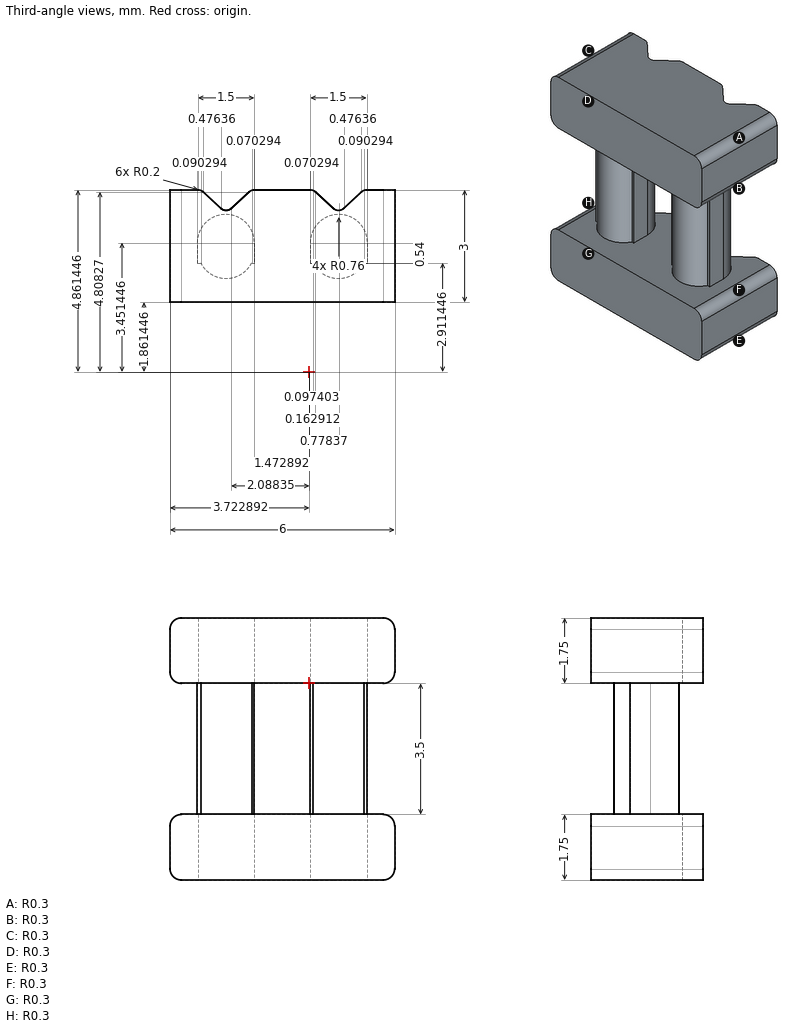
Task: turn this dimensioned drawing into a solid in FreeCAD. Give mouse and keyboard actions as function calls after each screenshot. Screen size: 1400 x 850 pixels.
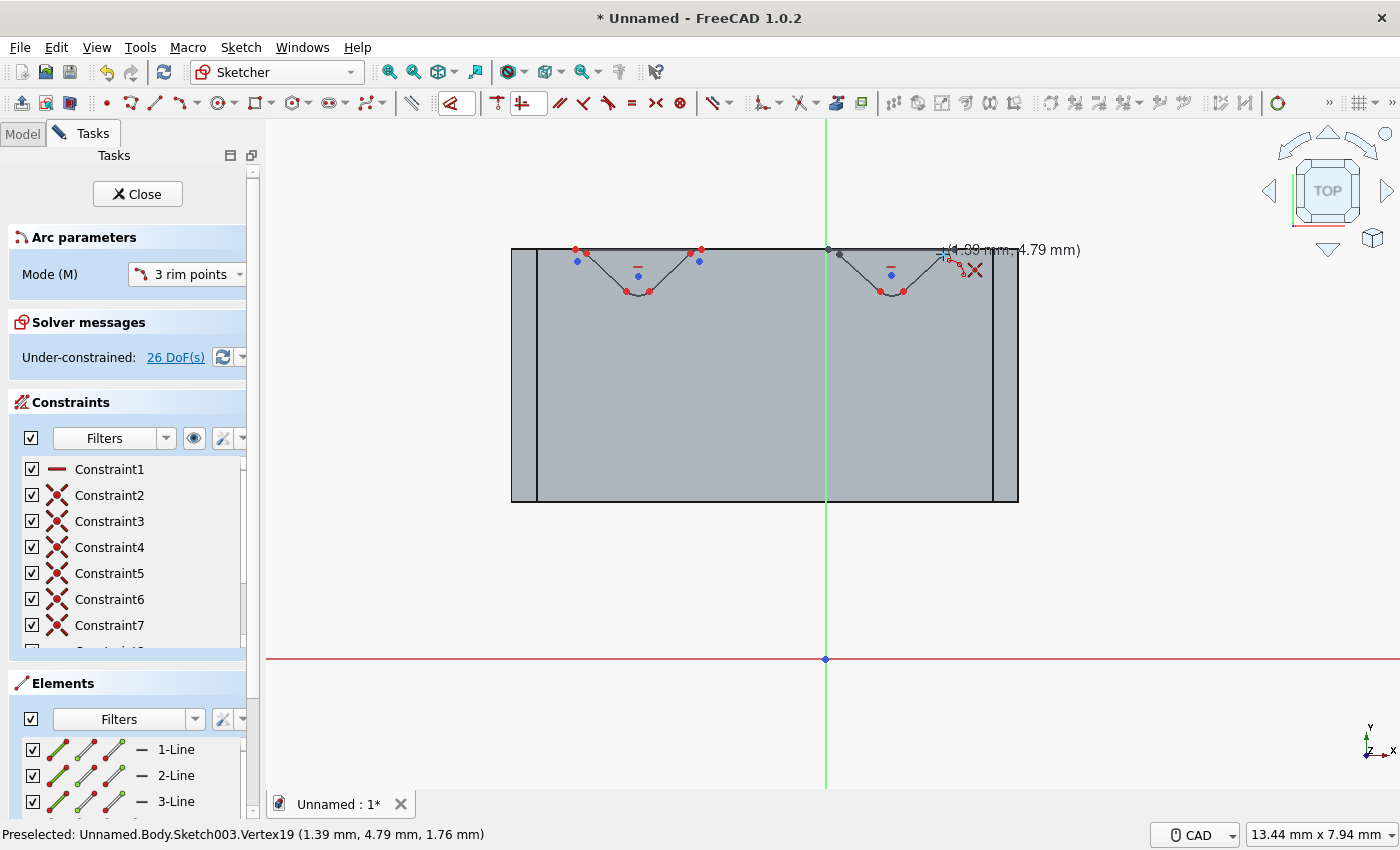
scroll(955, 249, up, 2)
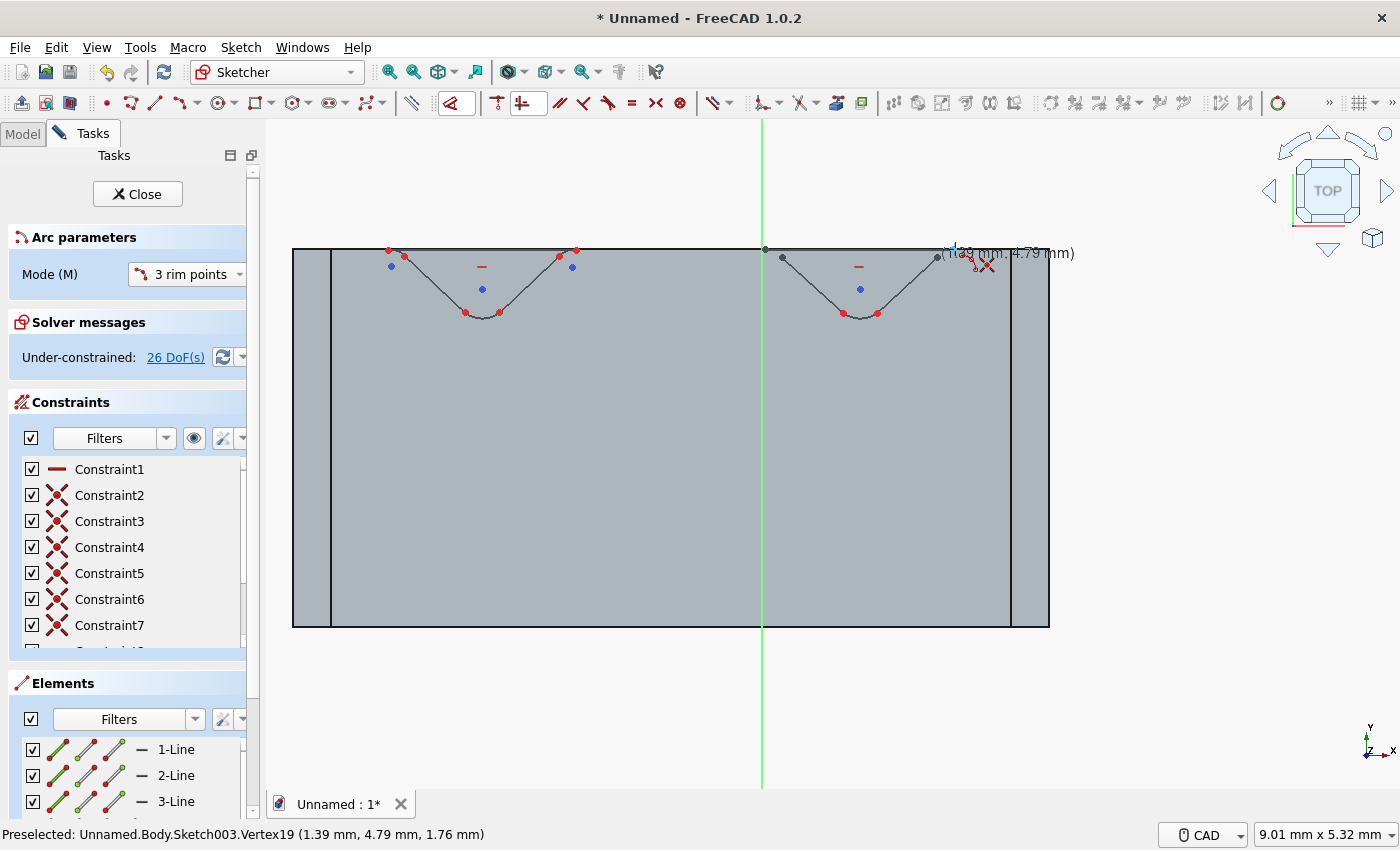
click(954, 250)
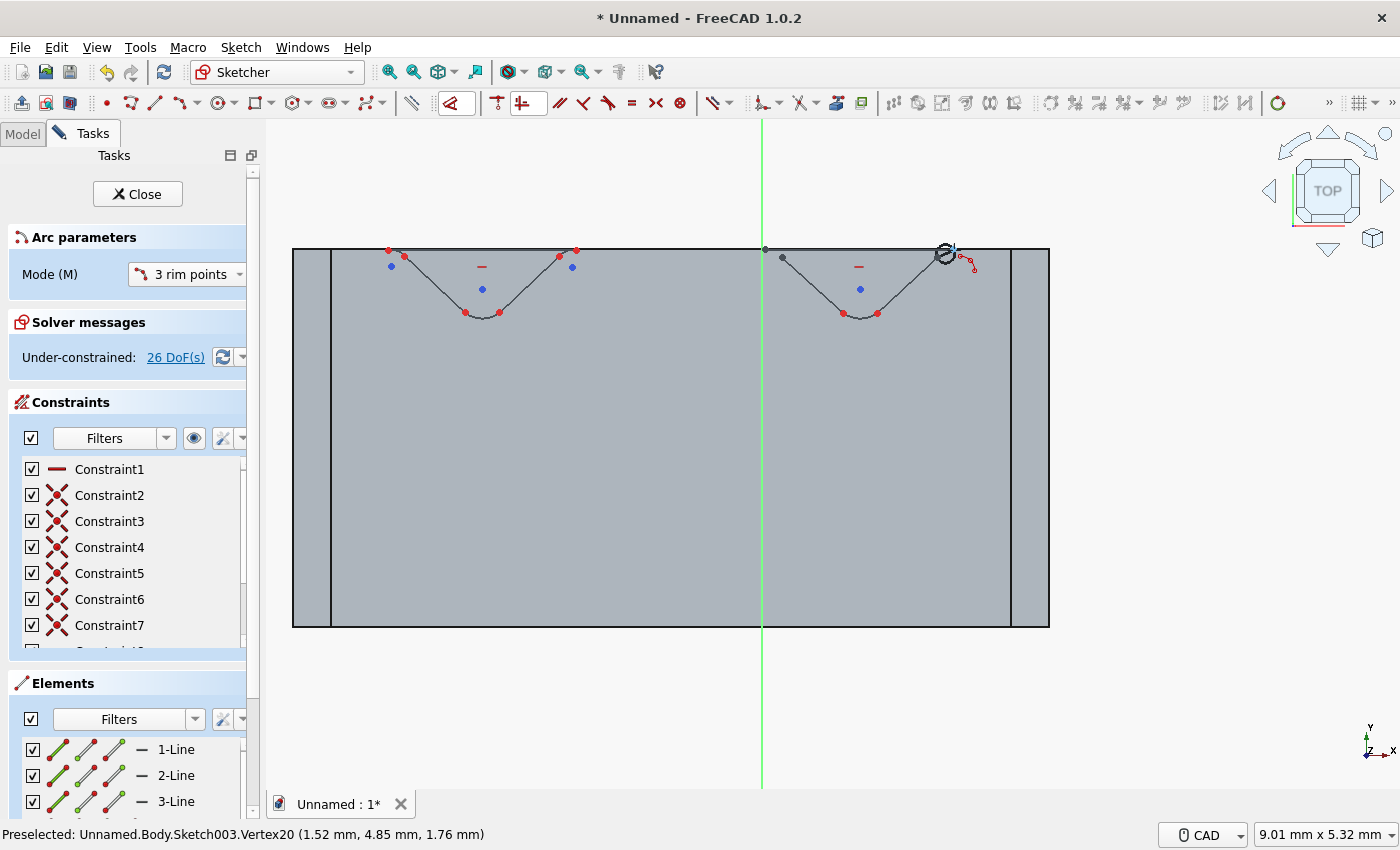
scroll(945, 251, up, 12)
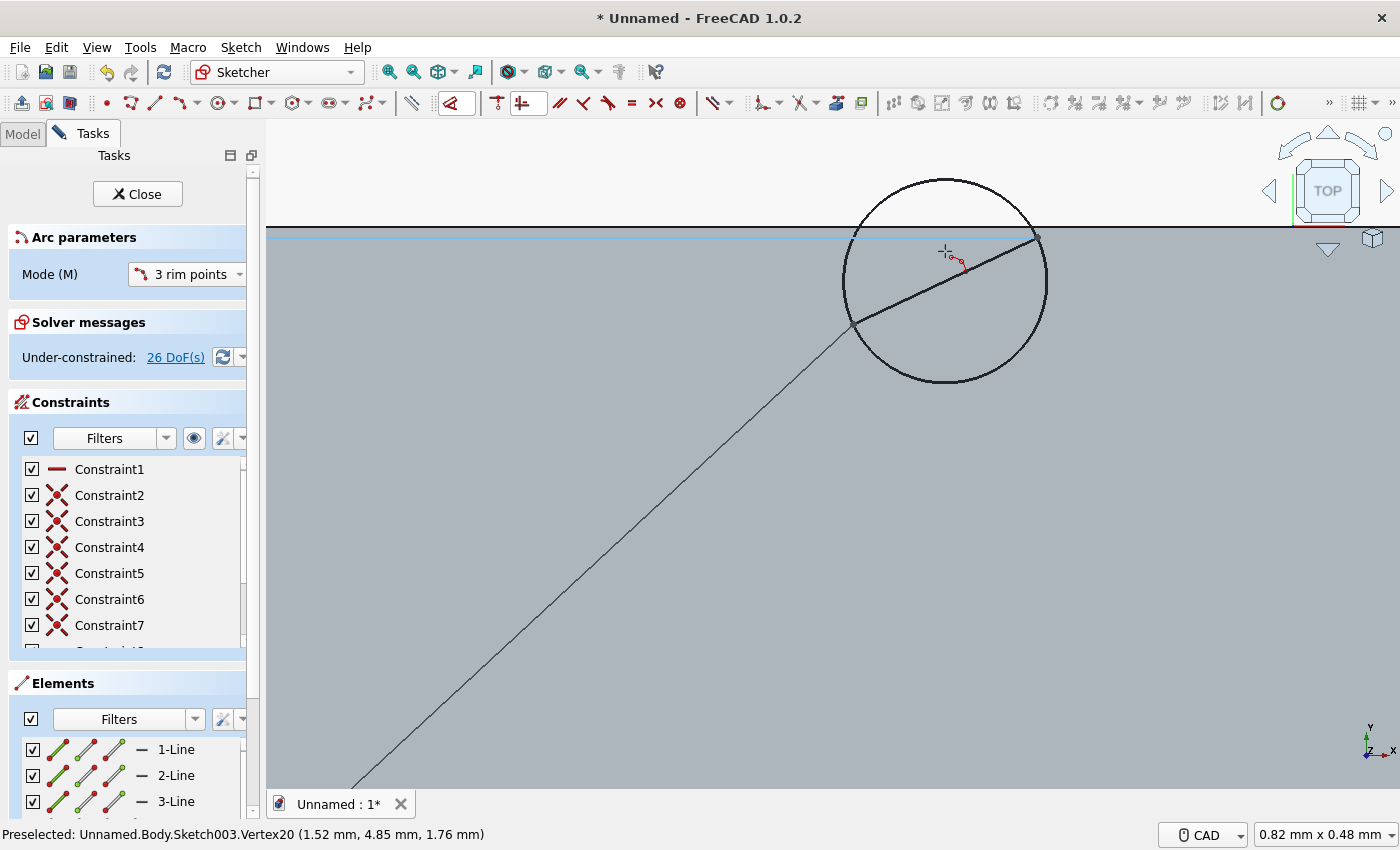
click(941, 246)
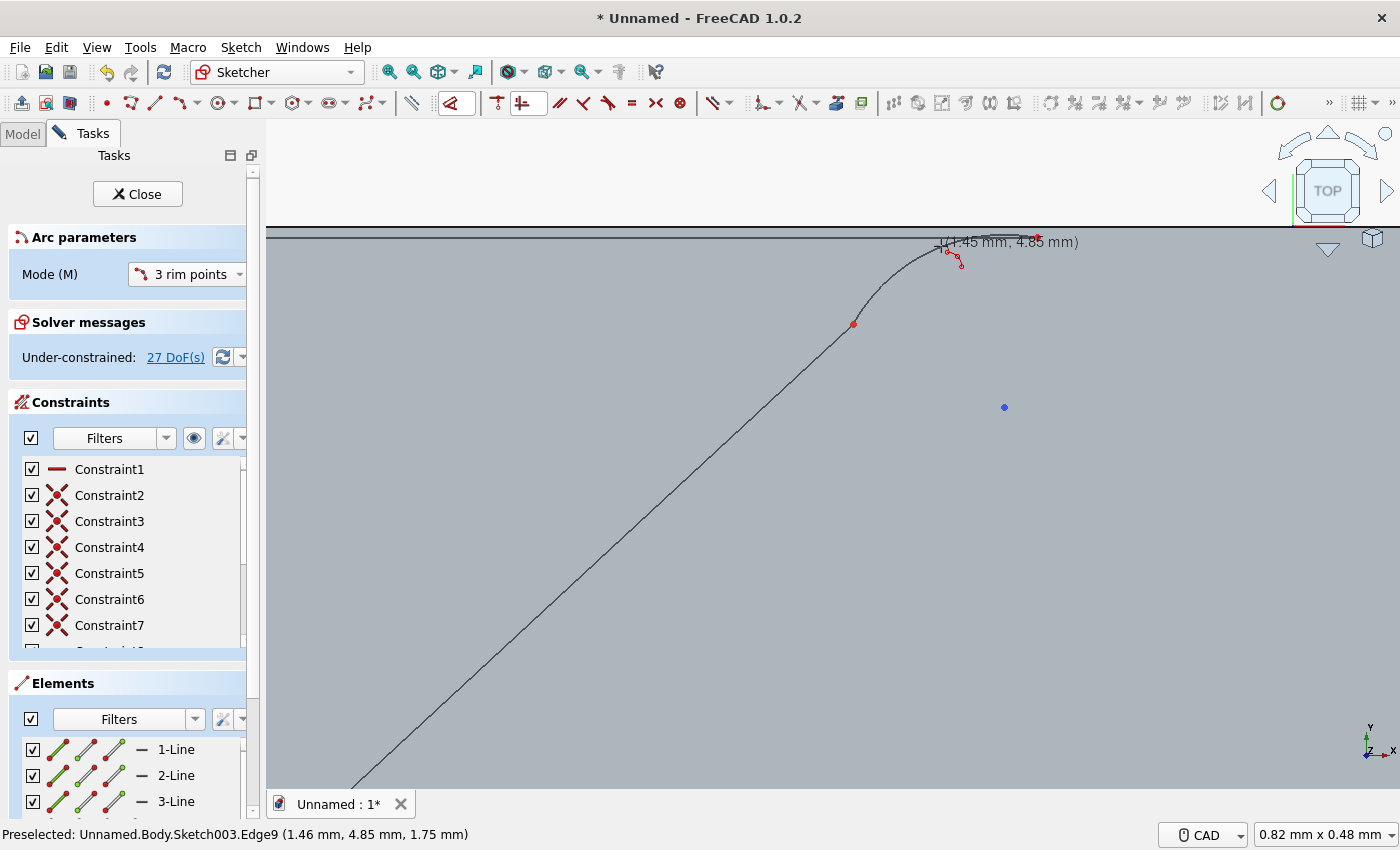
scroll(949, 250, down, 14)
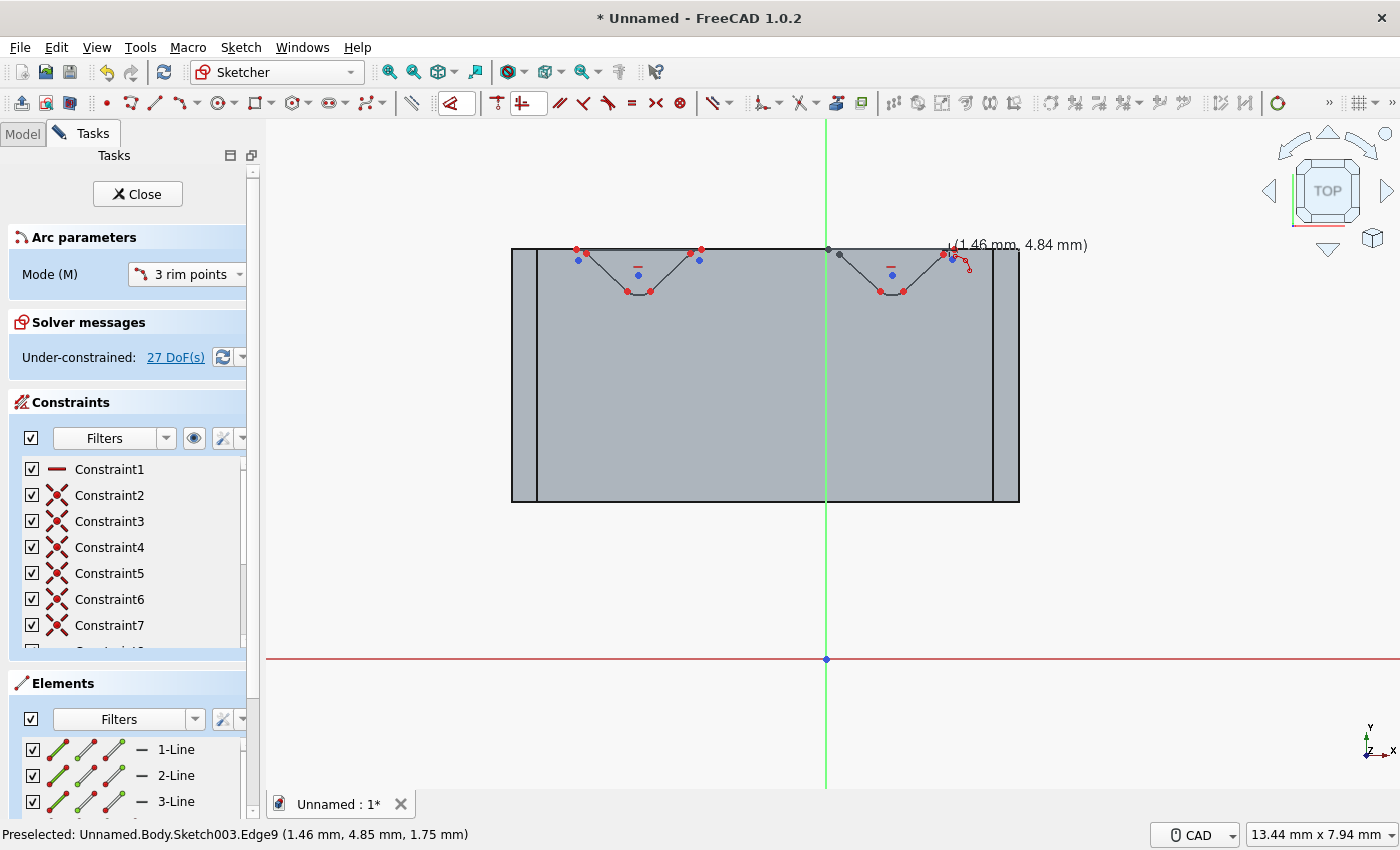
scroll(829, 249, up, 10)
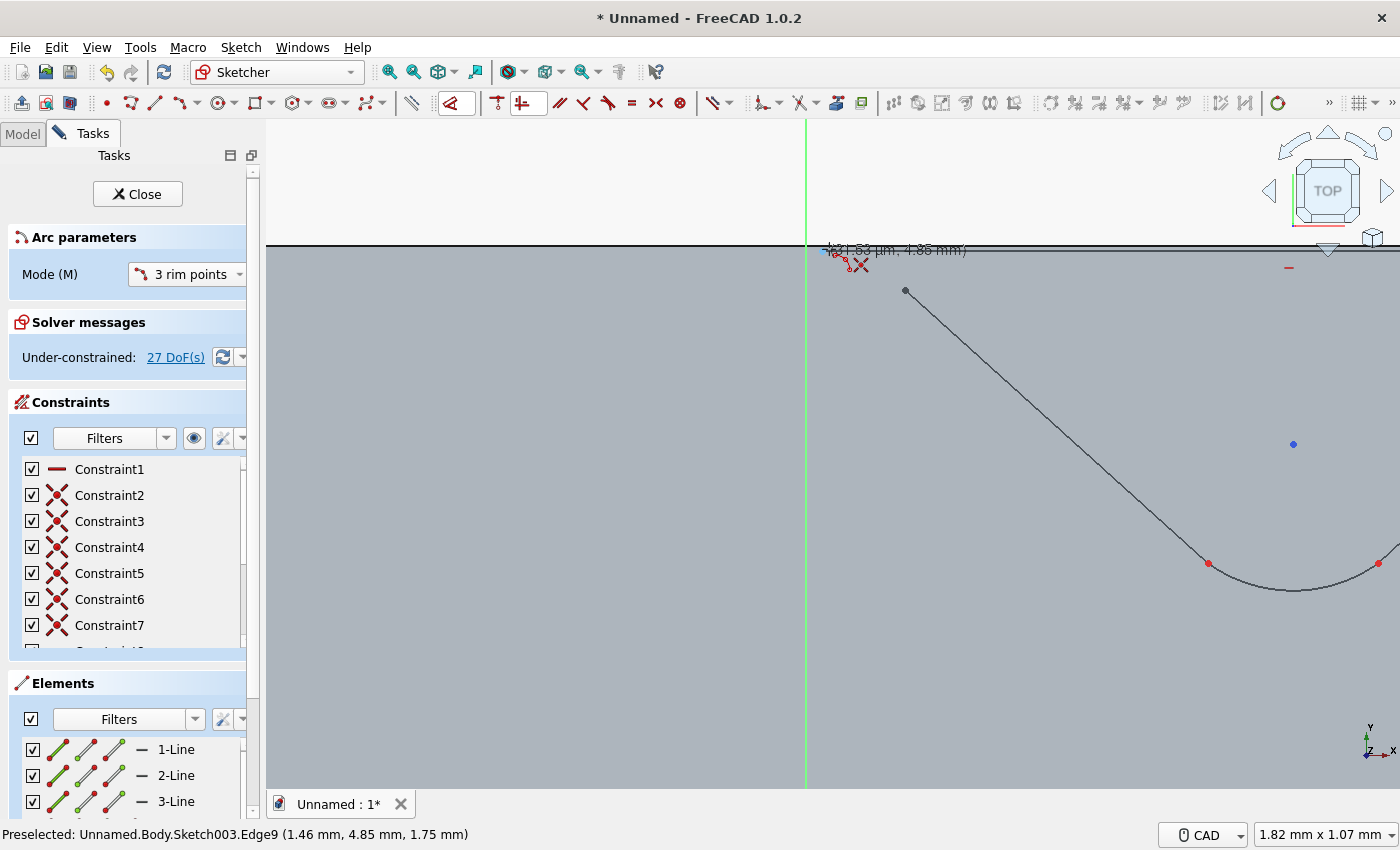
click(823, 251)
click(905, 290)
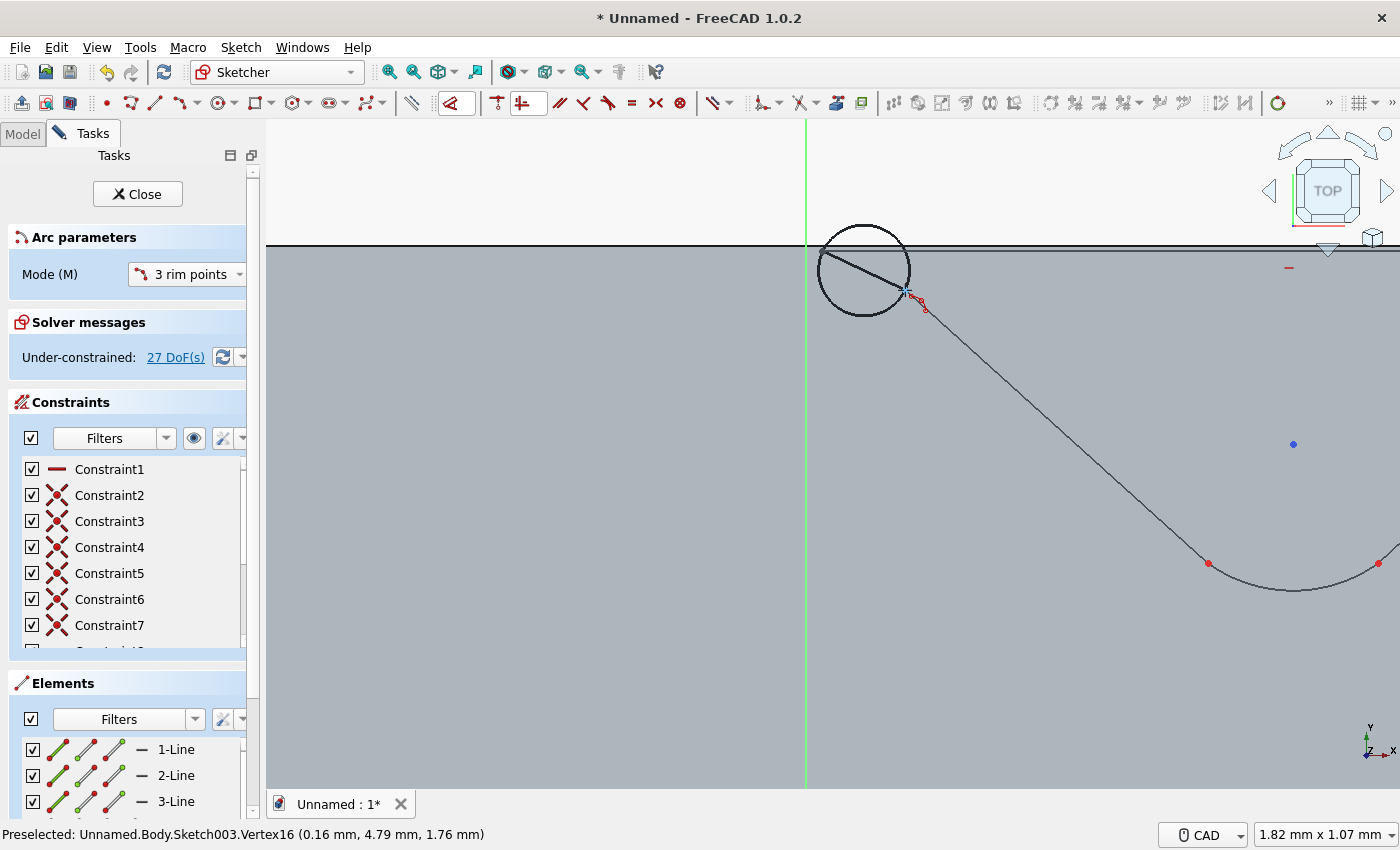
scroll(869, 255, up, 4)